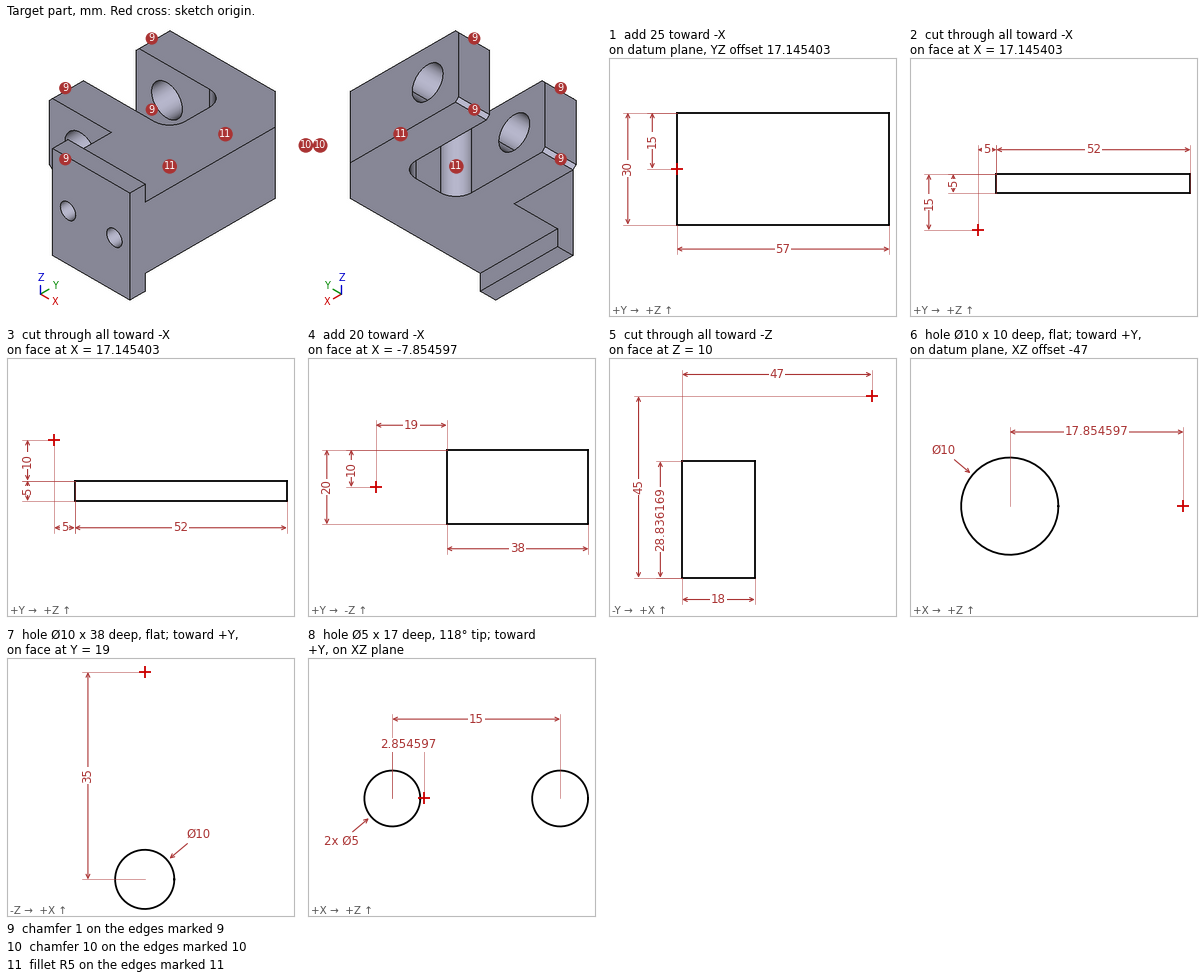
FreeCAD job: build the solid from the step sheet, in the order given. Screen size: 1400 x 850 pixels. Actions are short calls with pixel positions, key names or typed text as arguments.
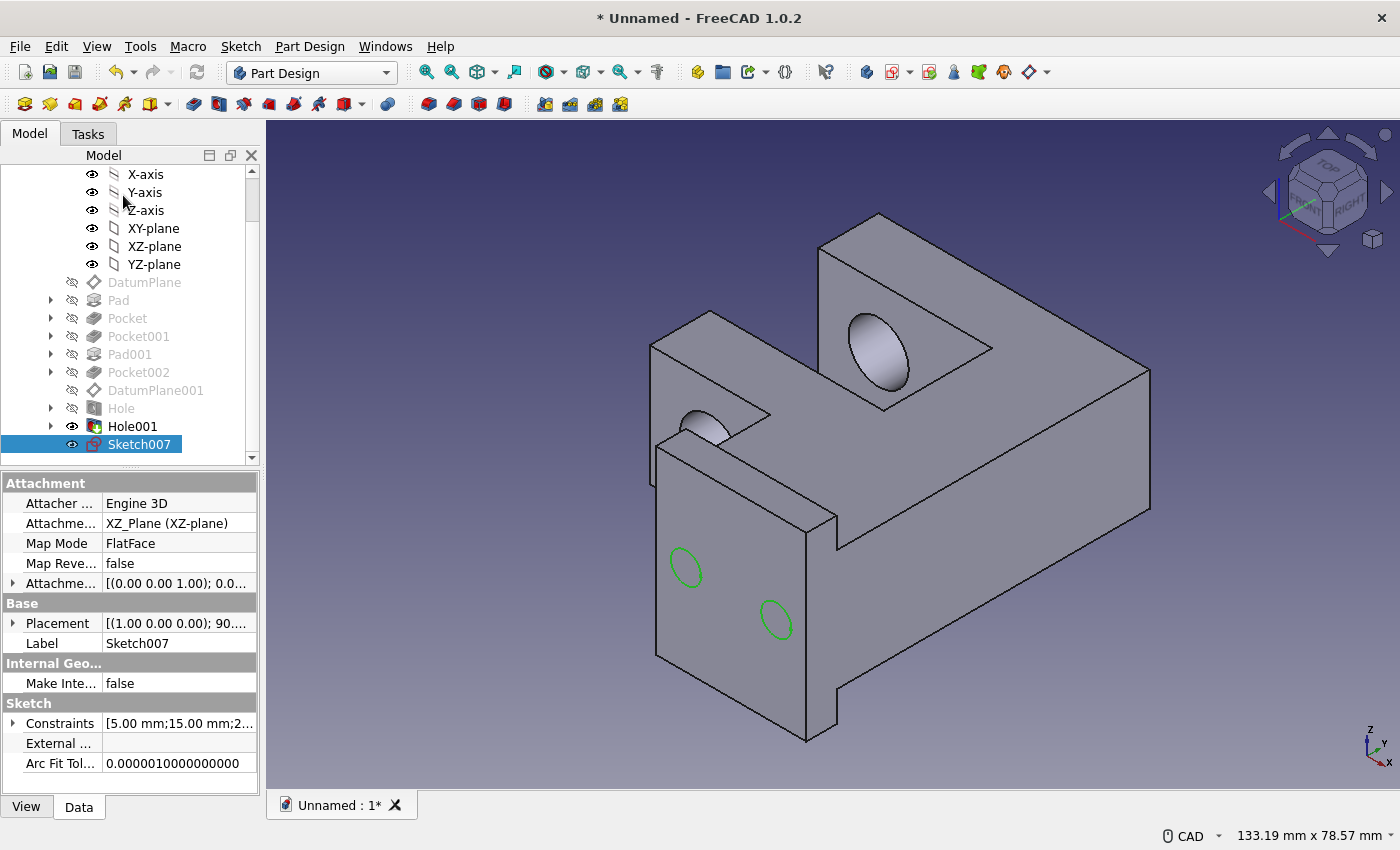
click(219, 104)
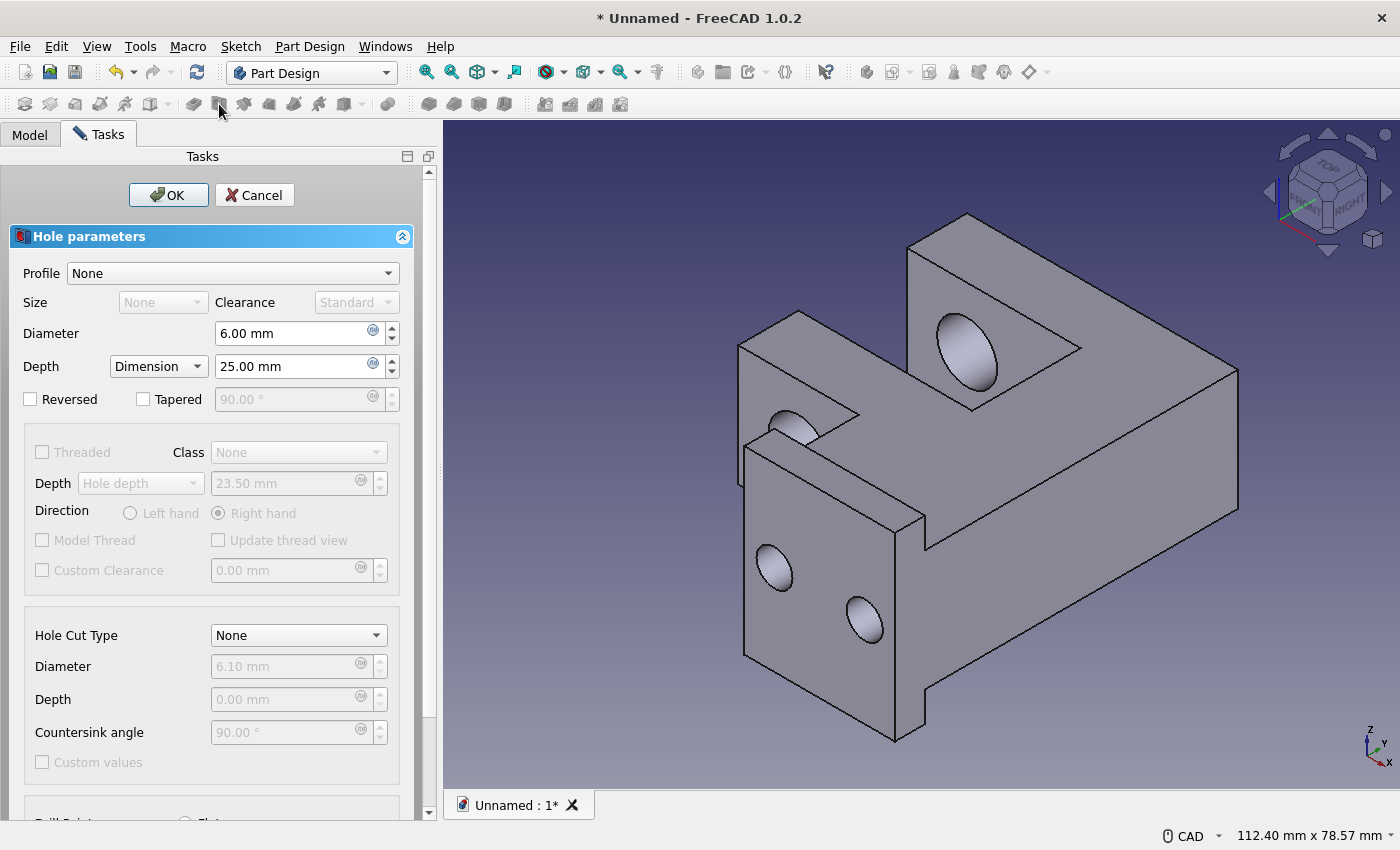
triple_click(300, 334)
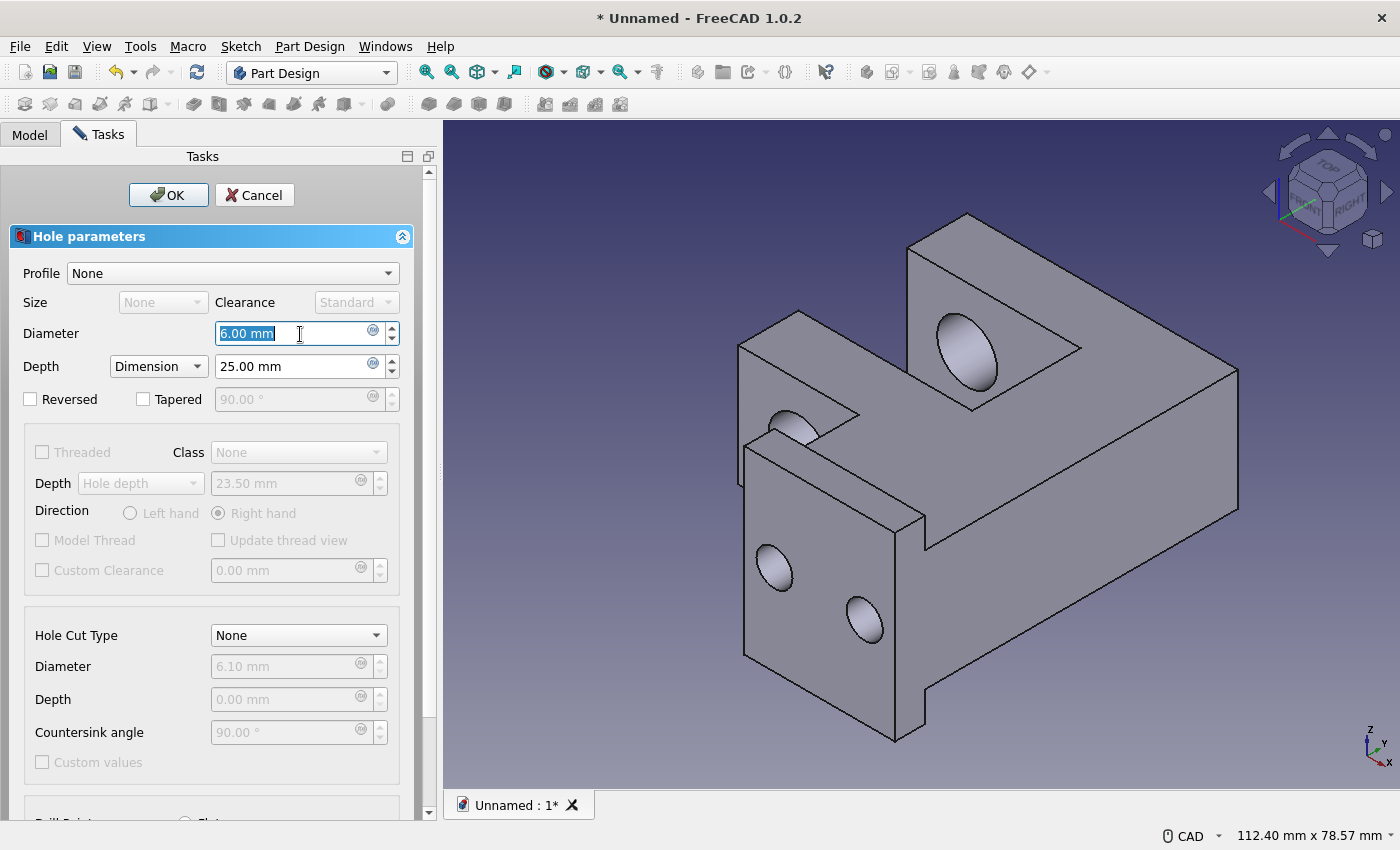
text(5)
key(Tab)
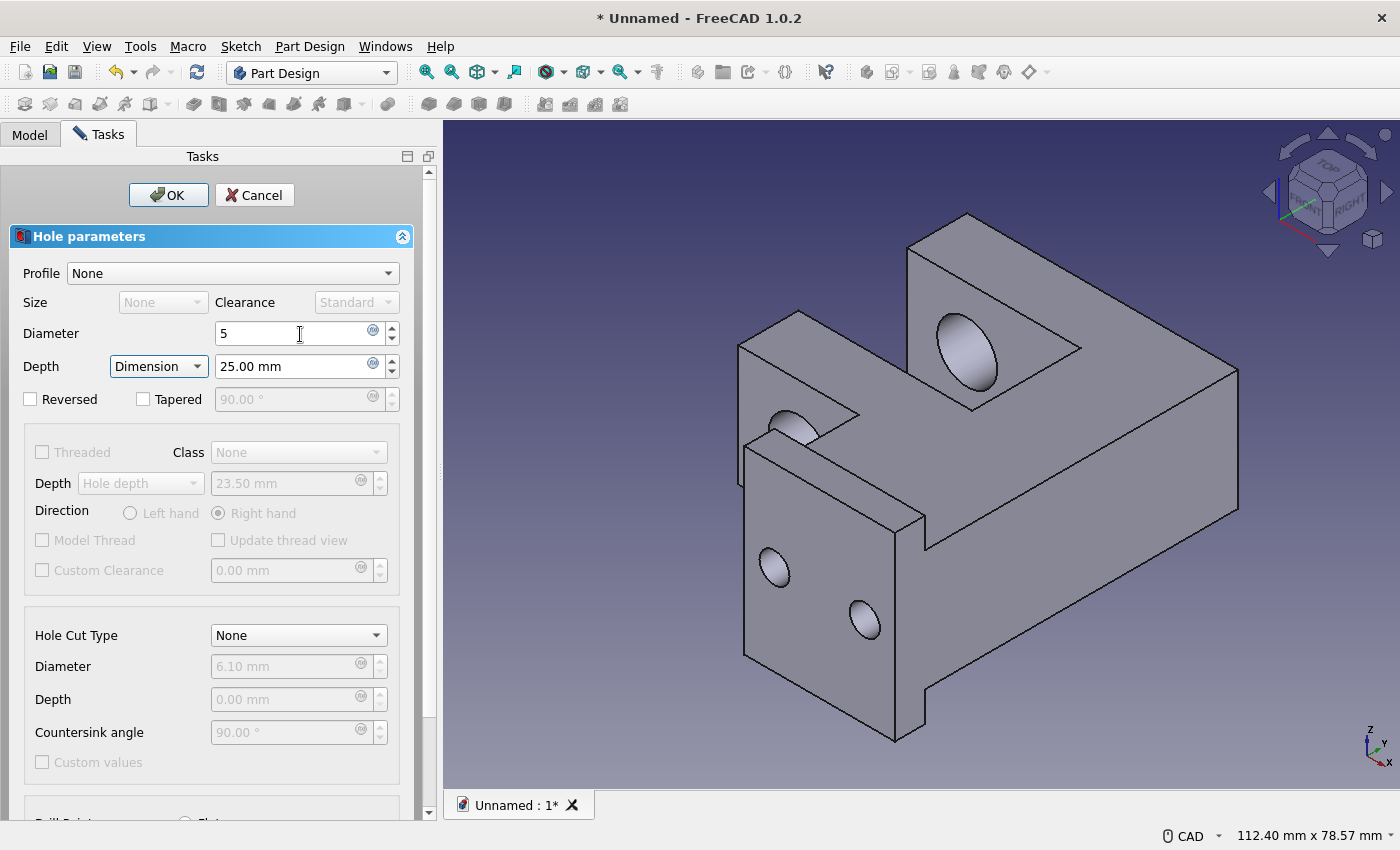
triple_click(300, 366)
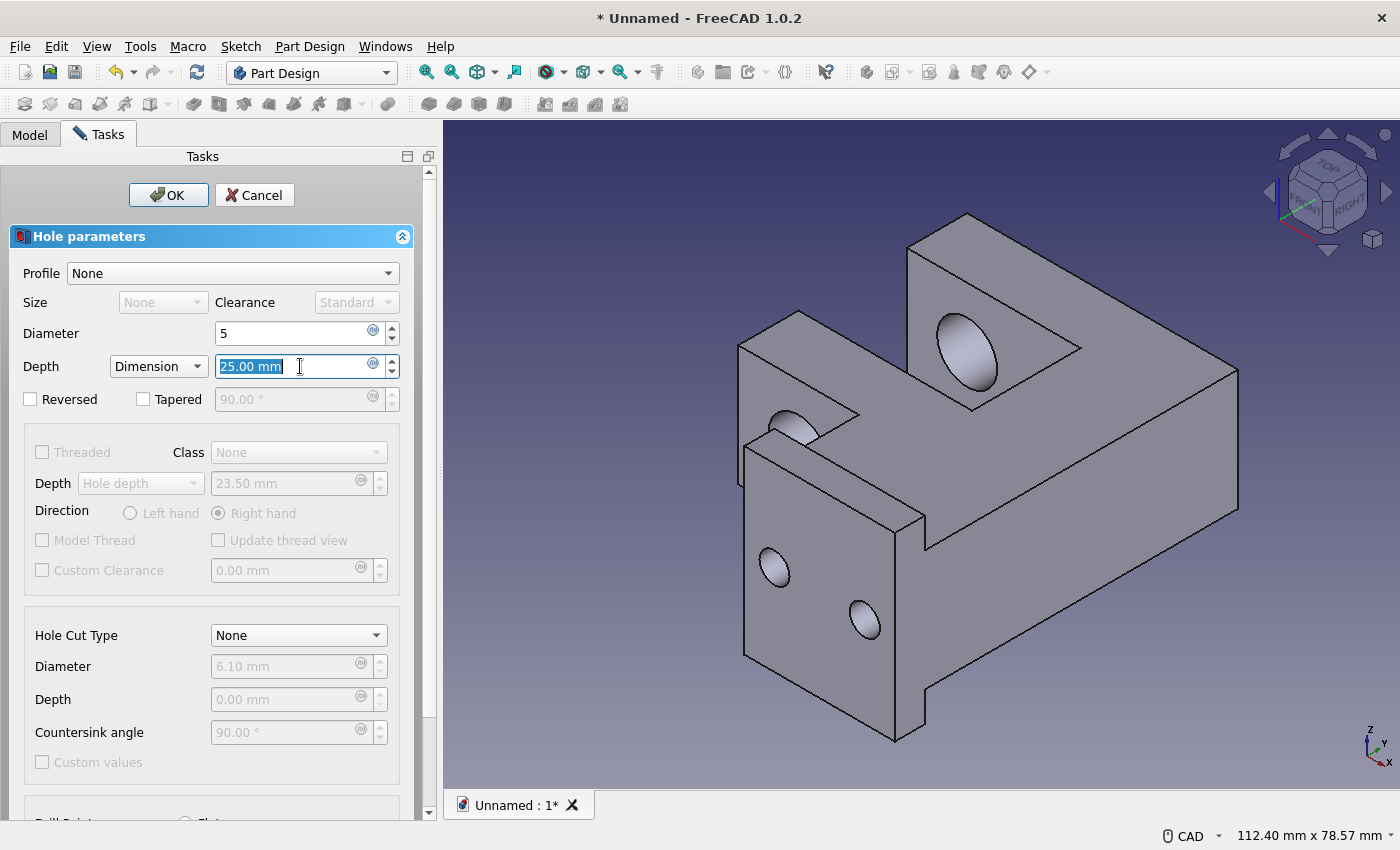
text(17)
key(Tab)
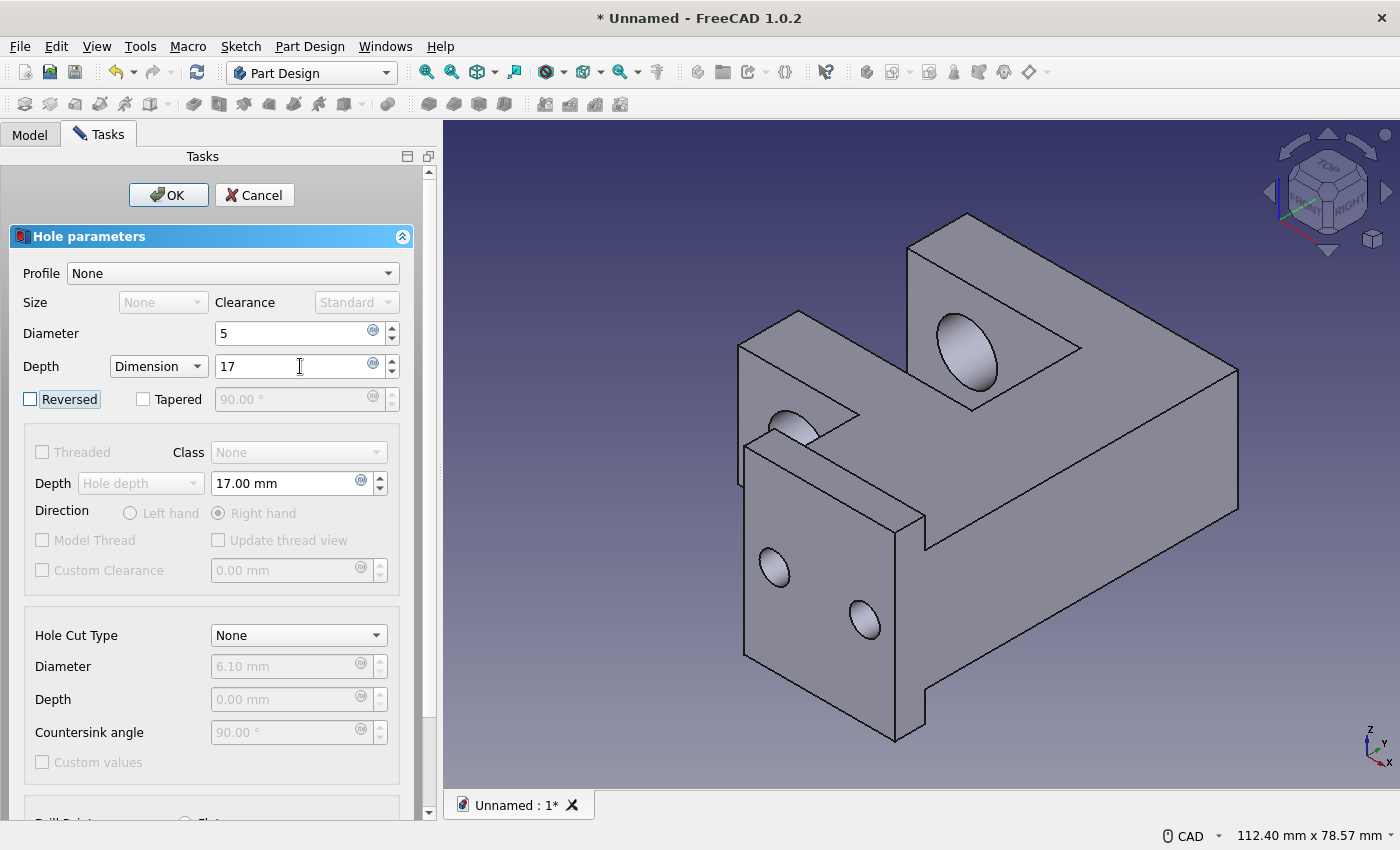
click(169, 195)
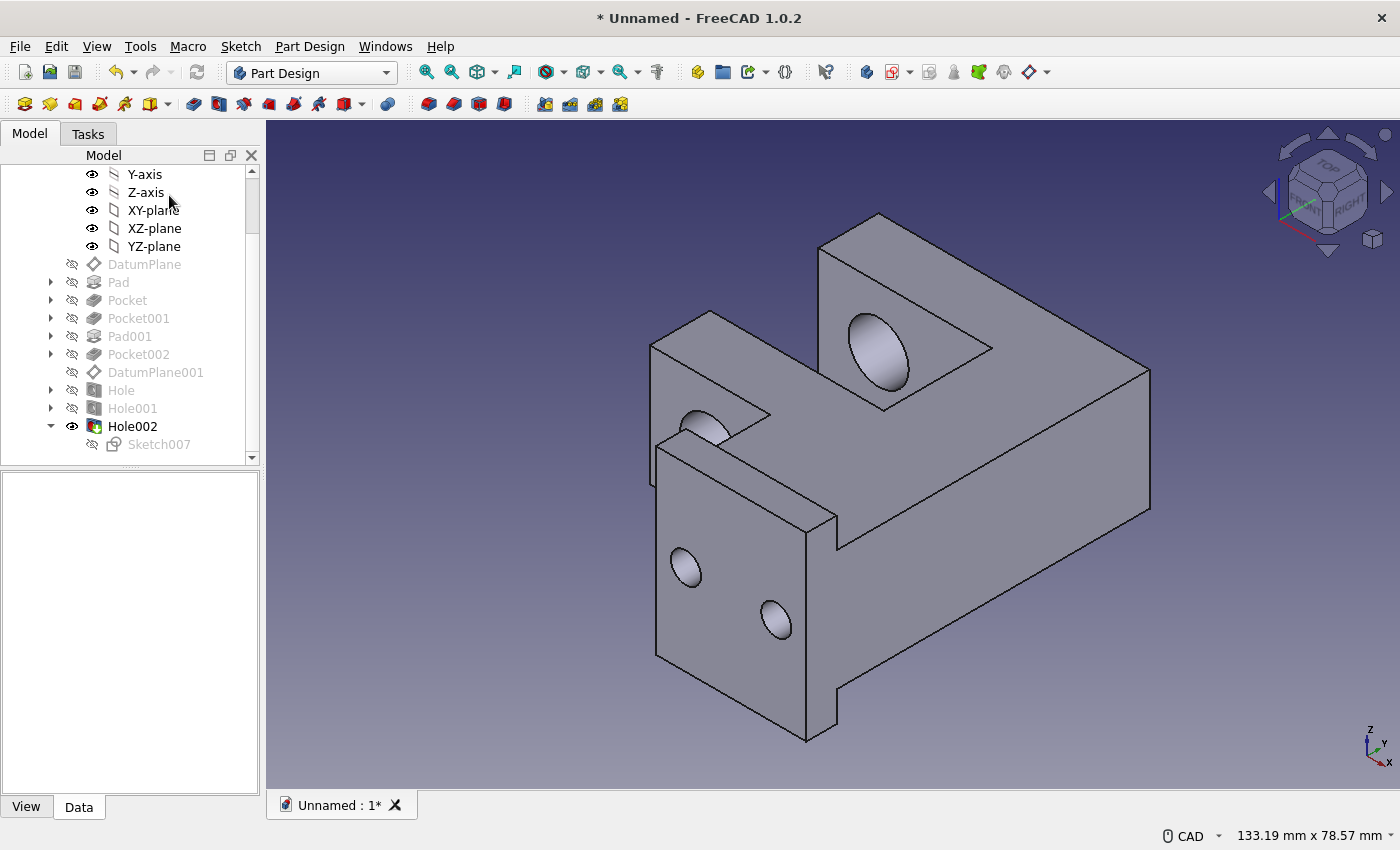
key(2)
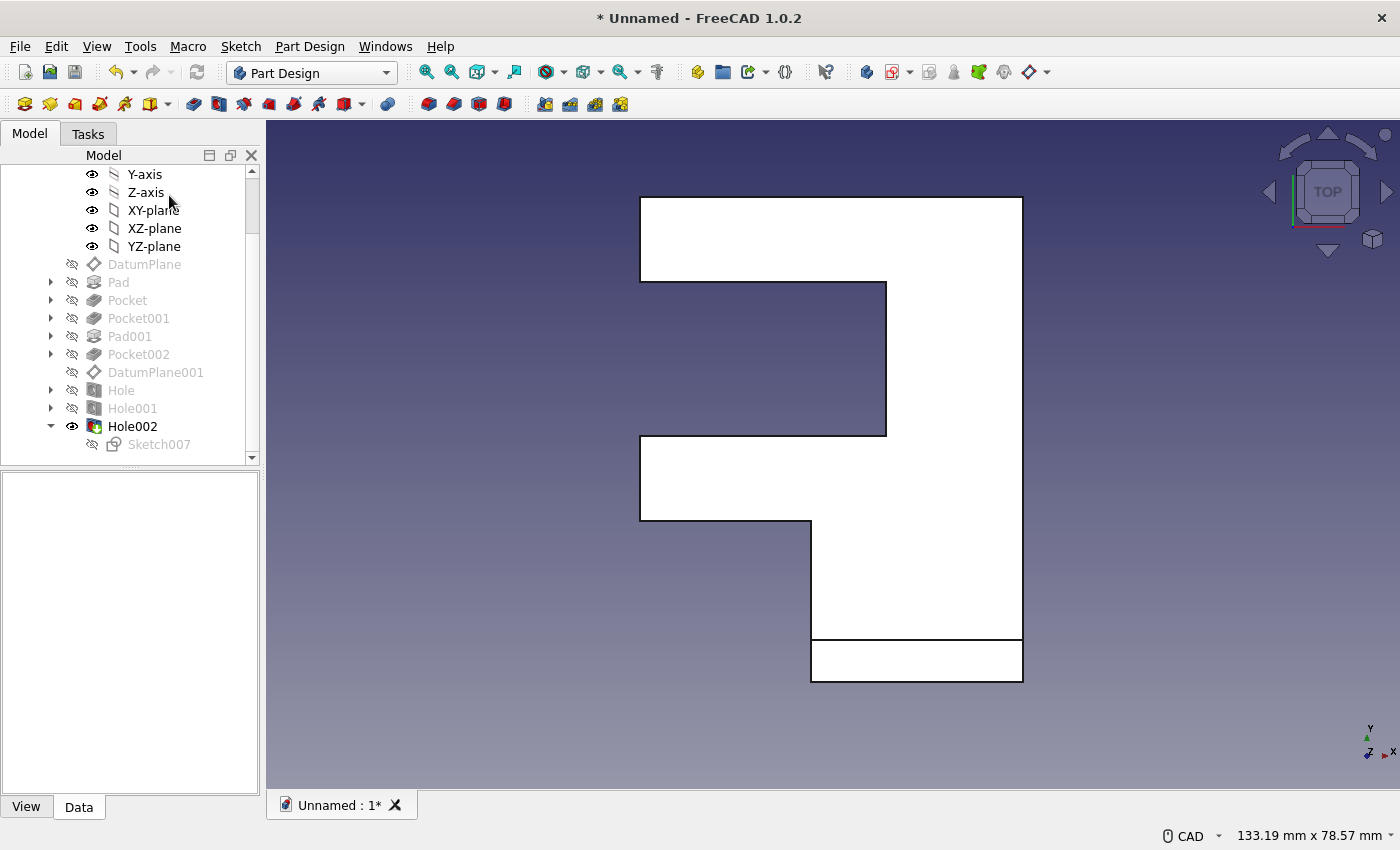
click(640, 477)